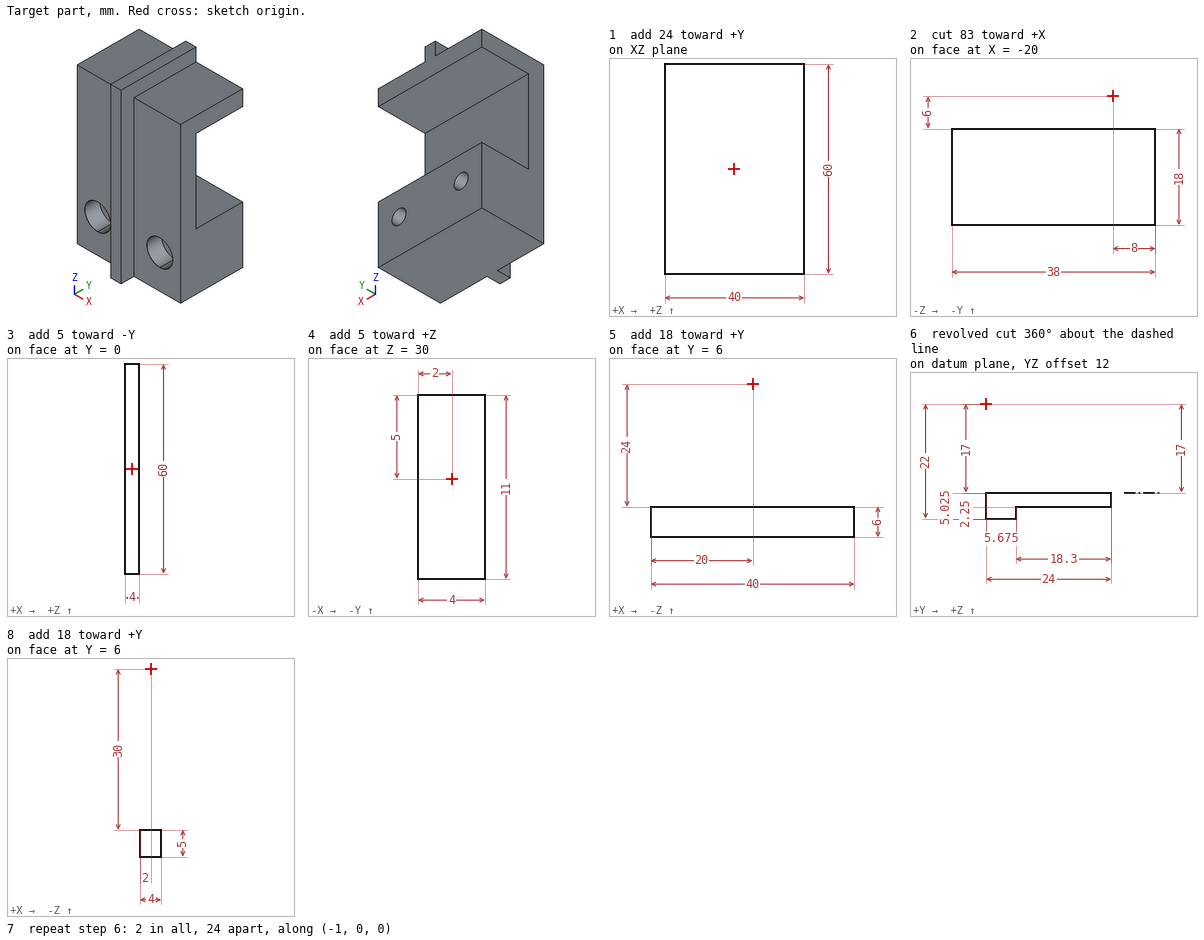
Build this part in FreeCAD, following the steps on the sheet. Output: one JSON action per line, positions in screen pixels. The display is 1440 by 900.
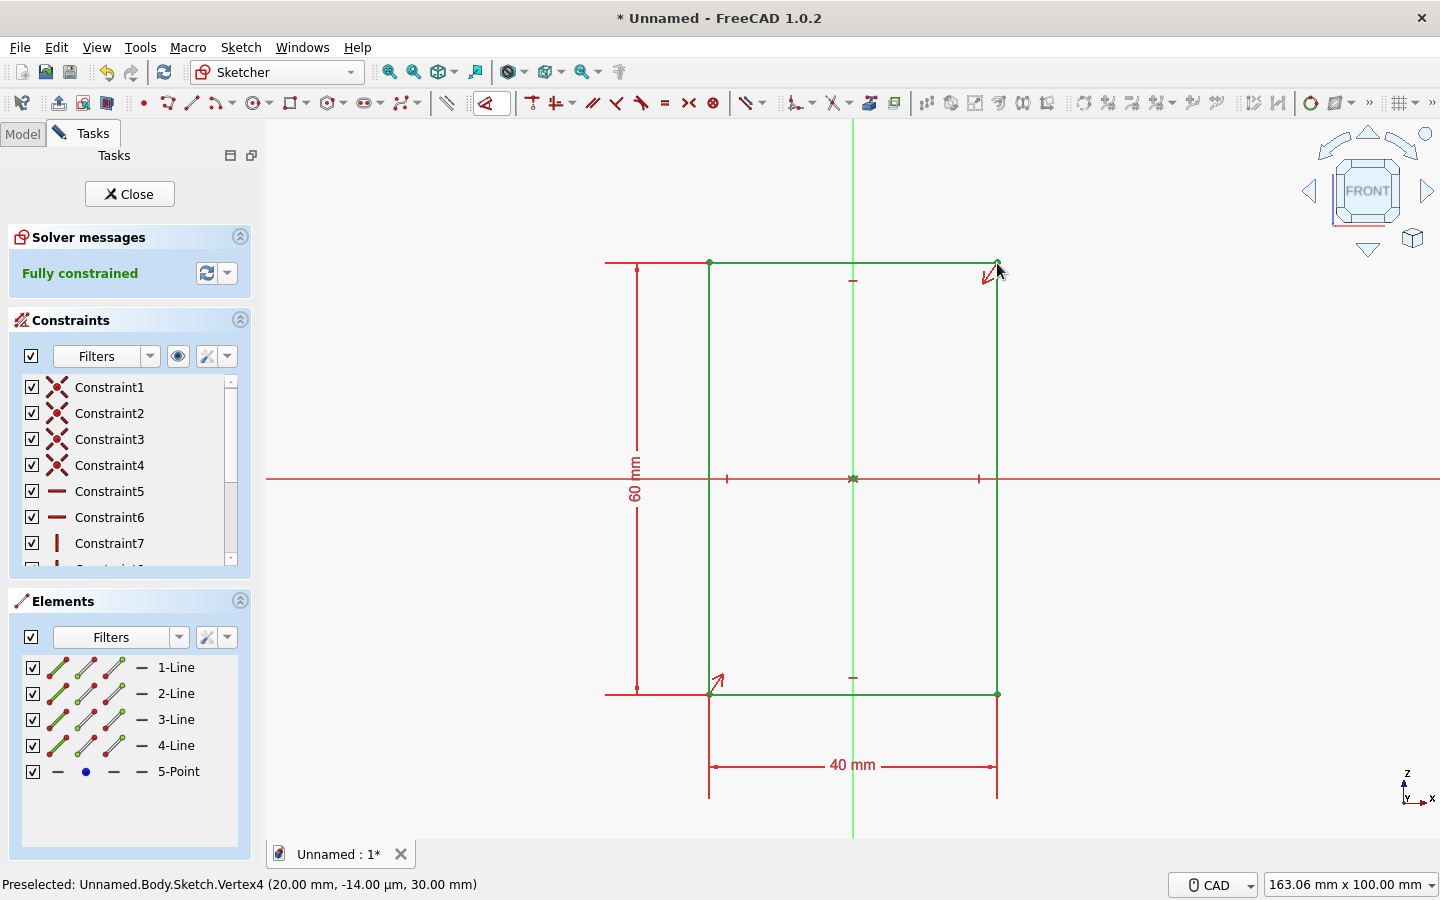
{"action": "left_click", "coordinate": [130, 194]}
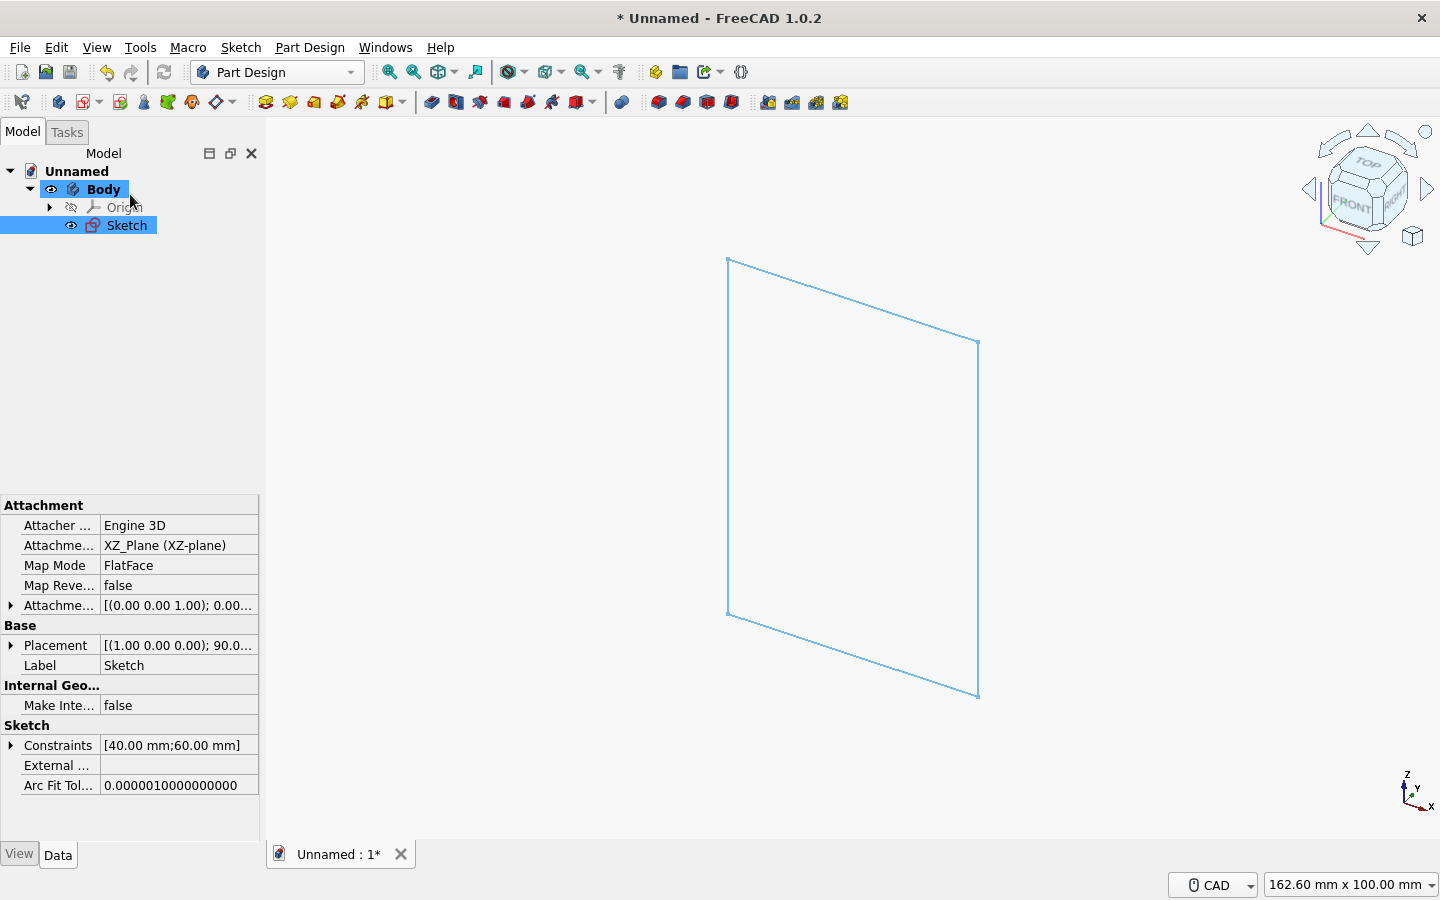
{"action": "left_click", "coordinate": [266, 102]}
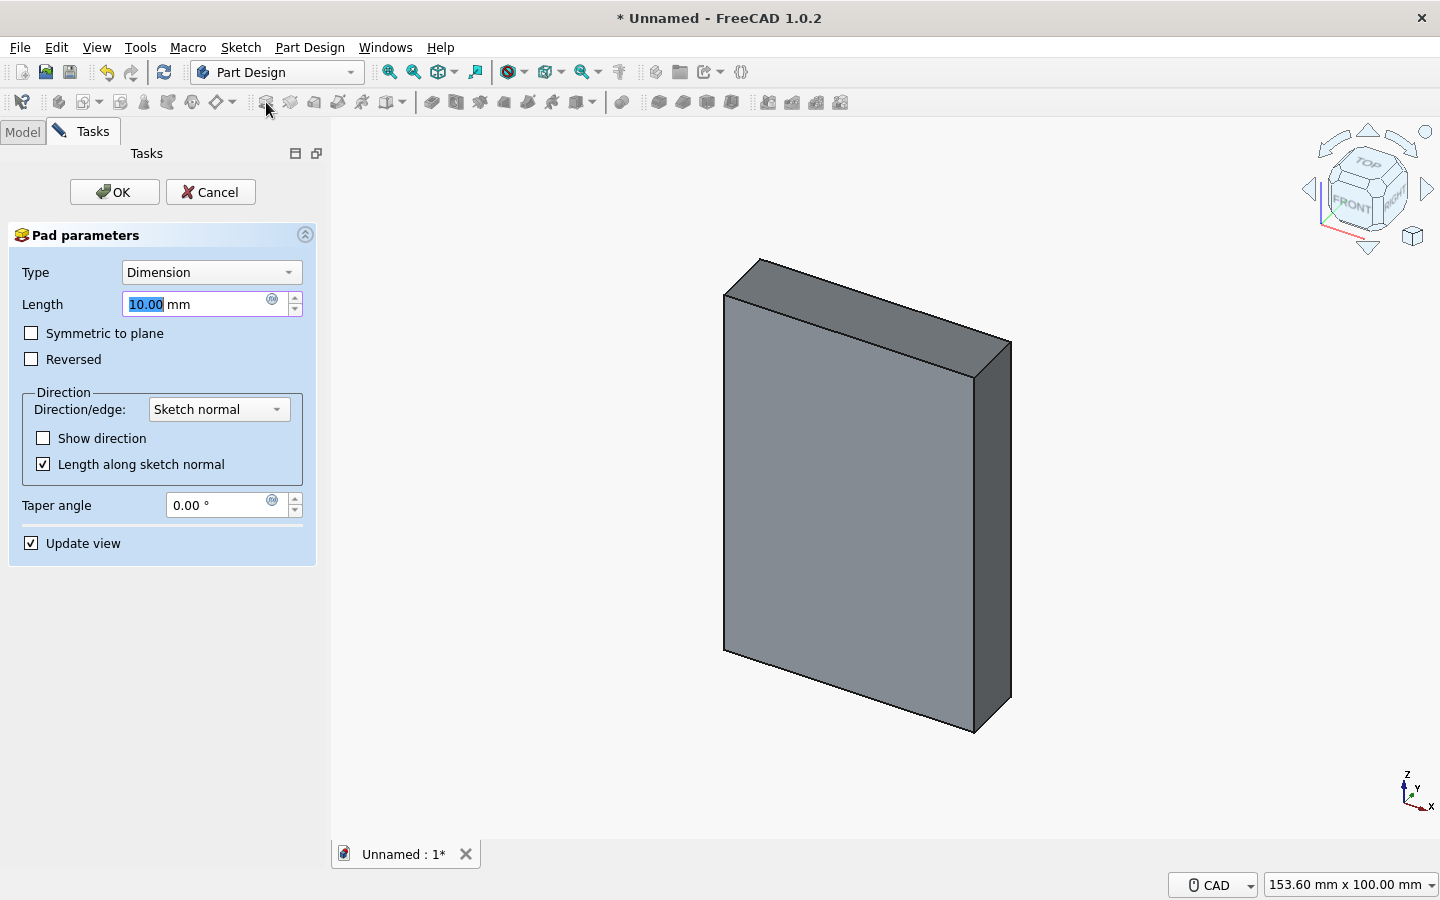
{"action": "type", "text": "24"}
{"action": "key", "text": "Tab"}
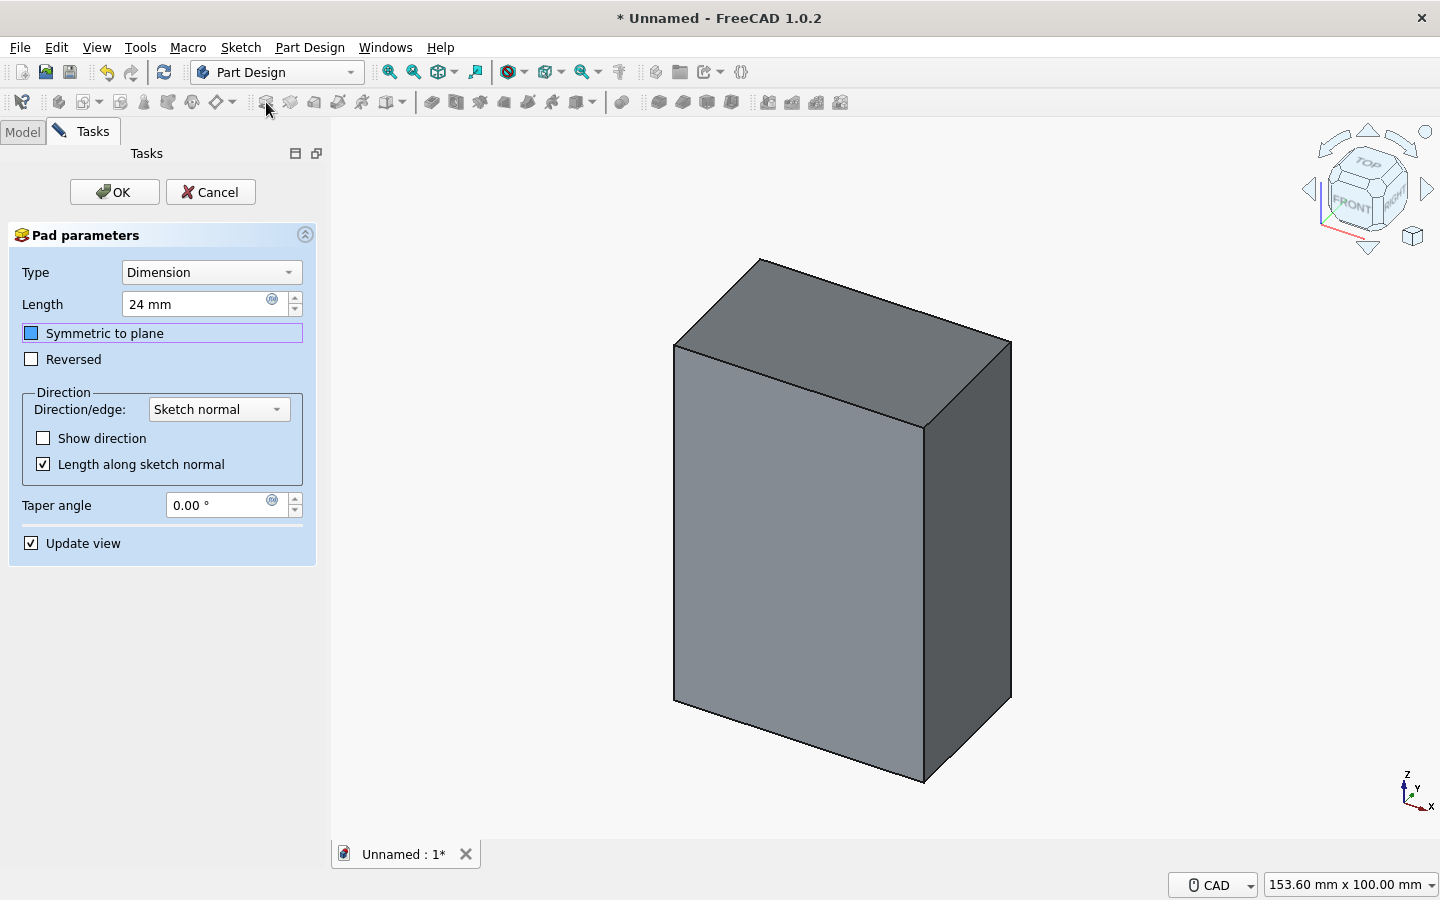
{"action": "left_click", "coordinate": [30, 359]}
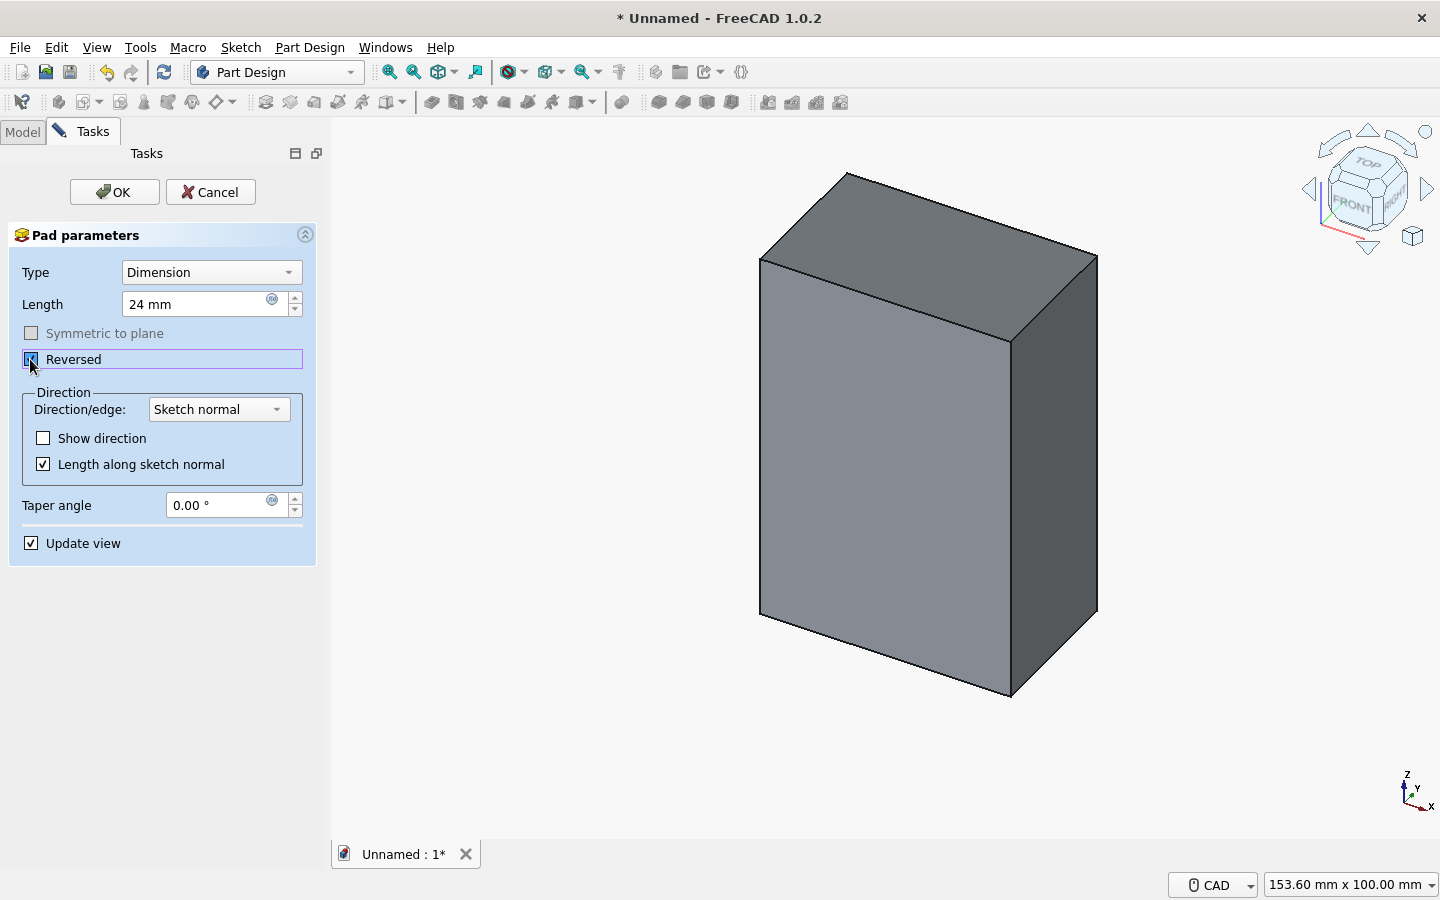
{"action": "left_click", "coordinate": [115, 192]}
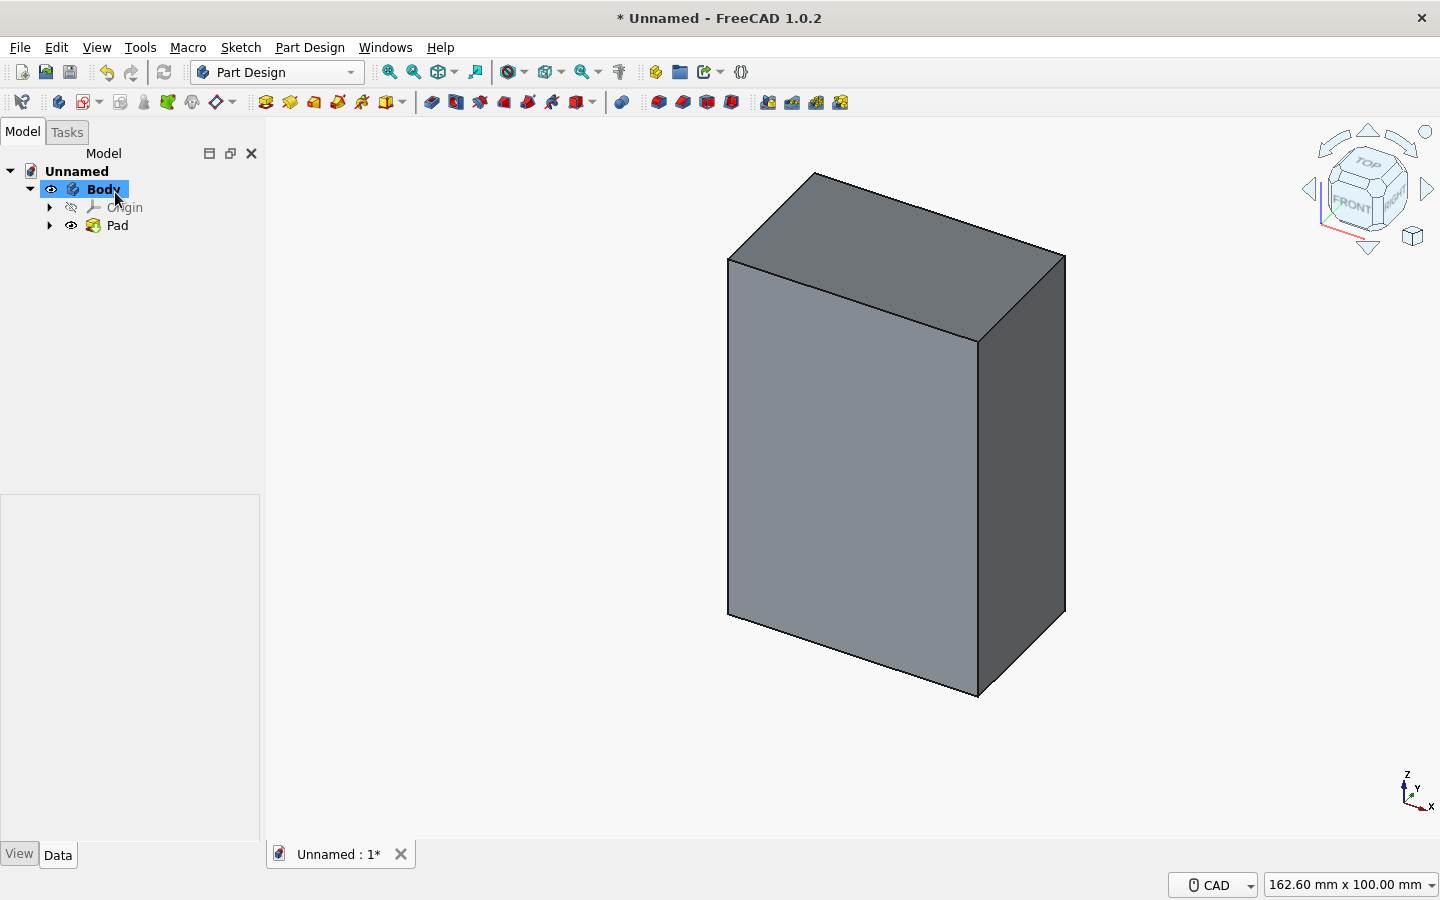
{"action": "key", "text": "6"}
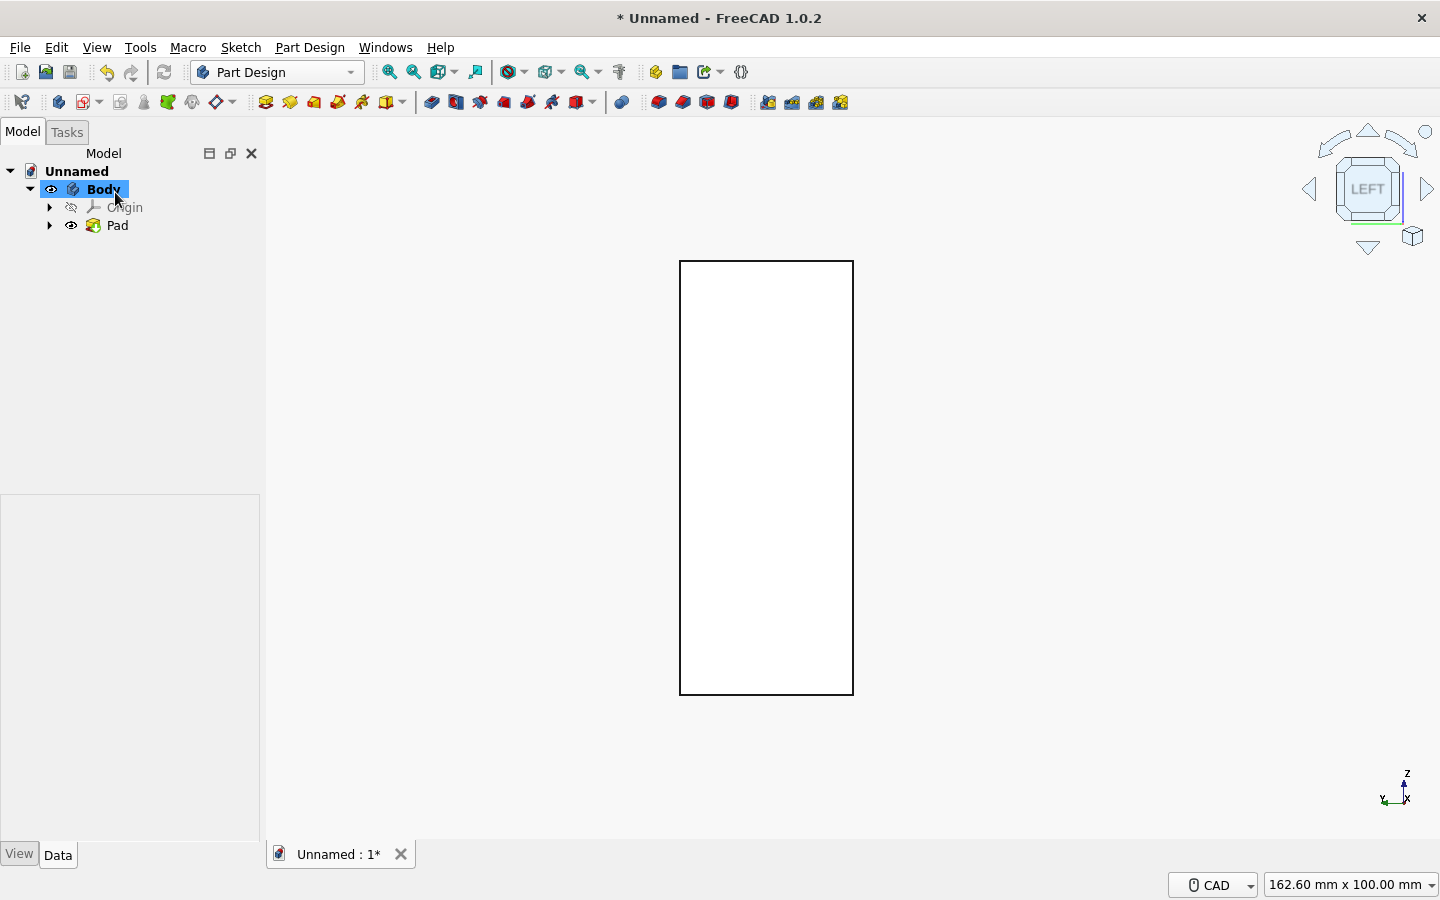
{"action": "left_click", "coordinate": [766, 353]}